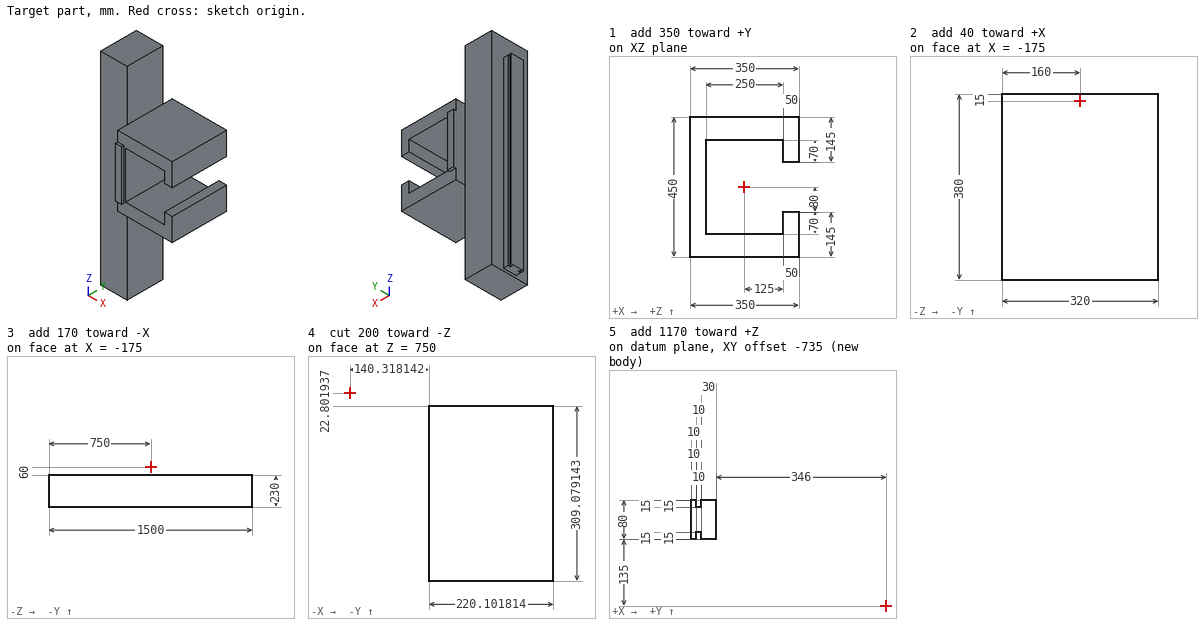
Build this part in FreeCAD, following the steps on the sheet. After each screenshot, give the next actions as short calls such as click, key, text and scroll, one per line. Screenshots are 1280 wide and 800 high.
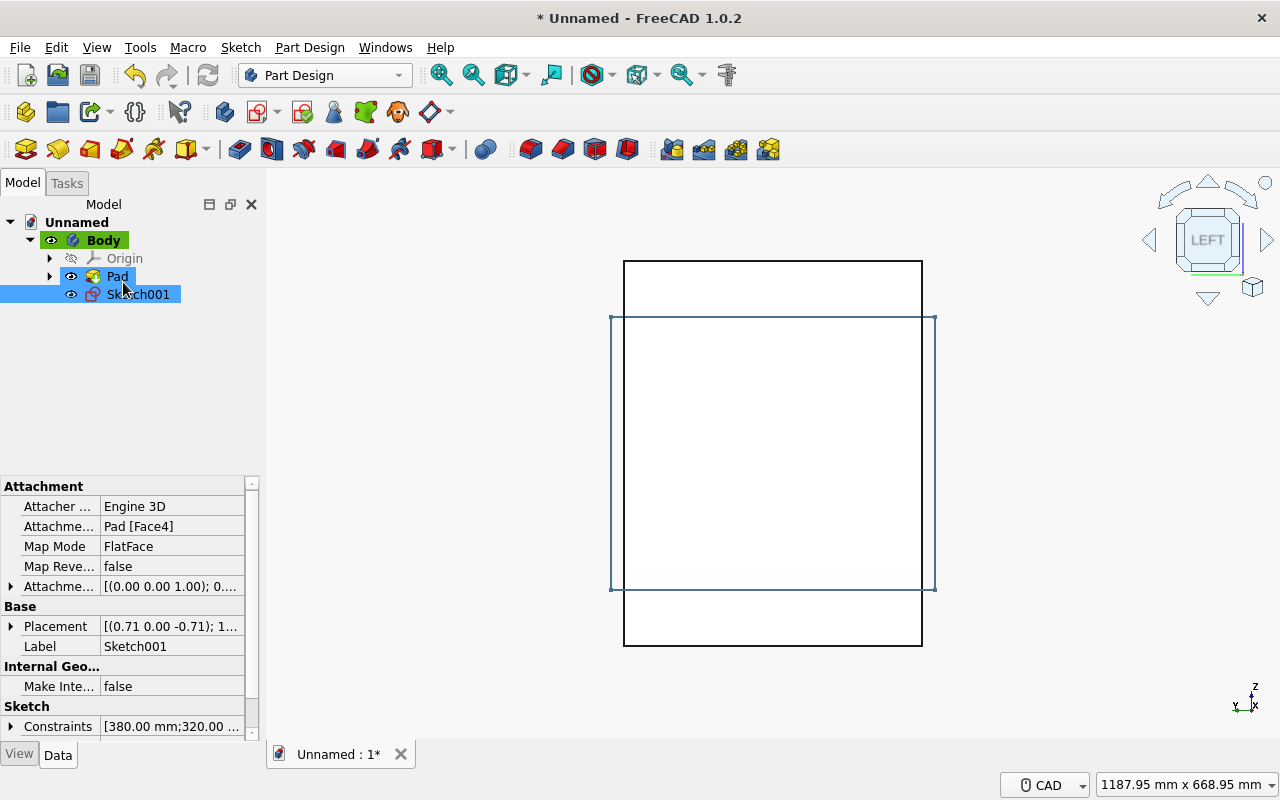
click(26, 150)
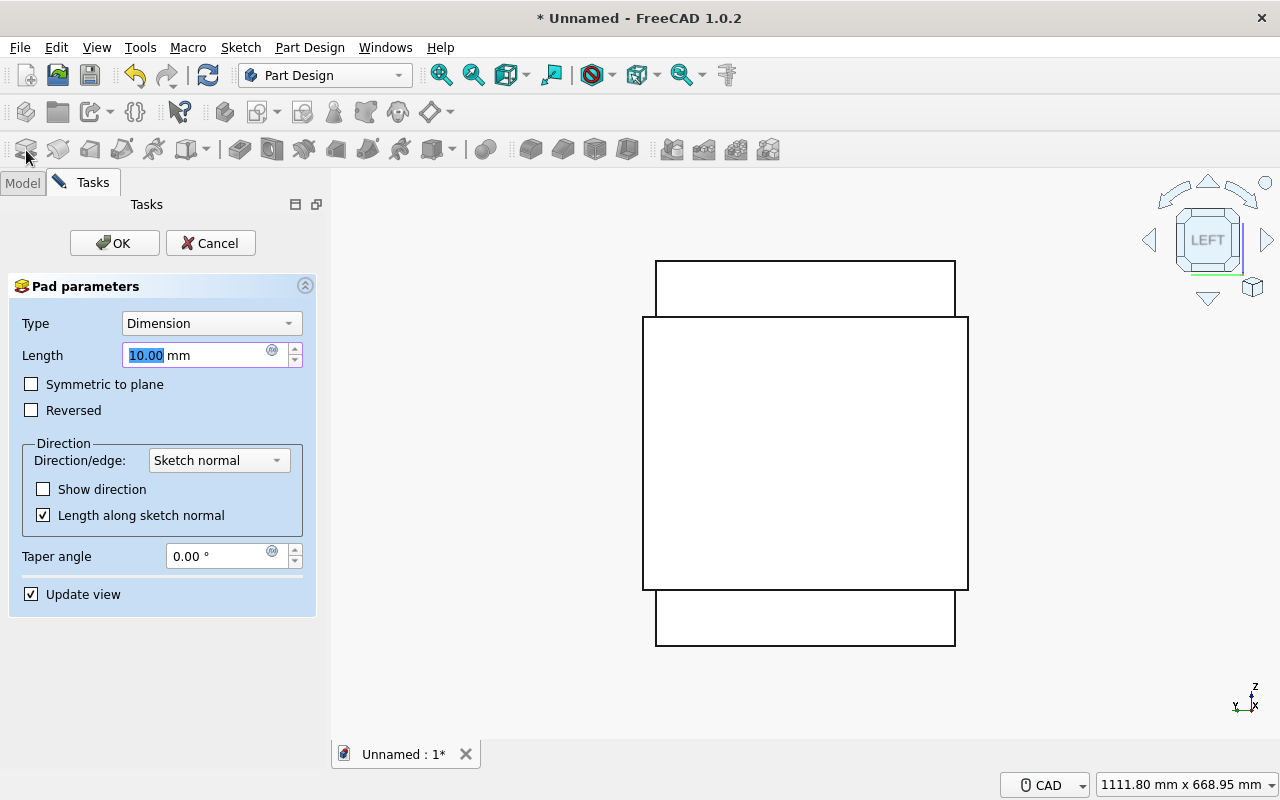
text(40)
key(Tab)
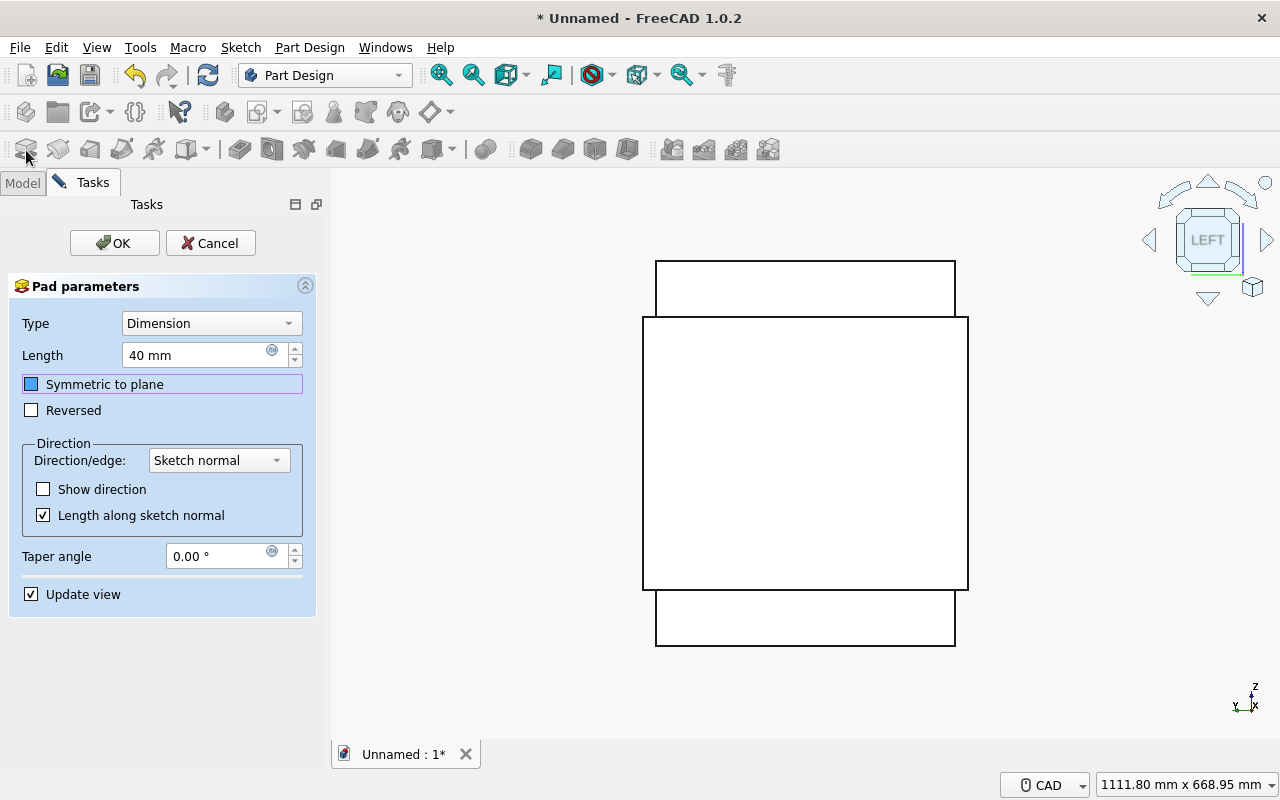
click(30, 410)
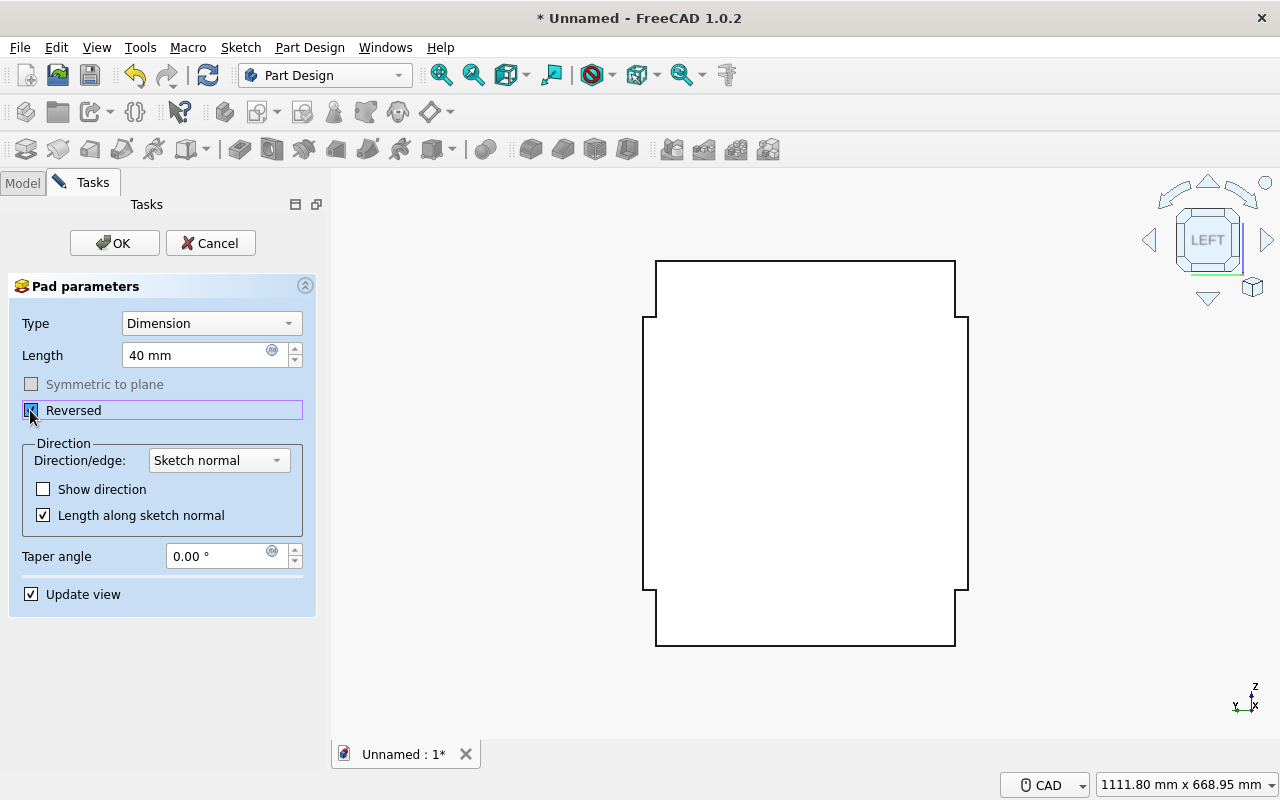
click(115, 243)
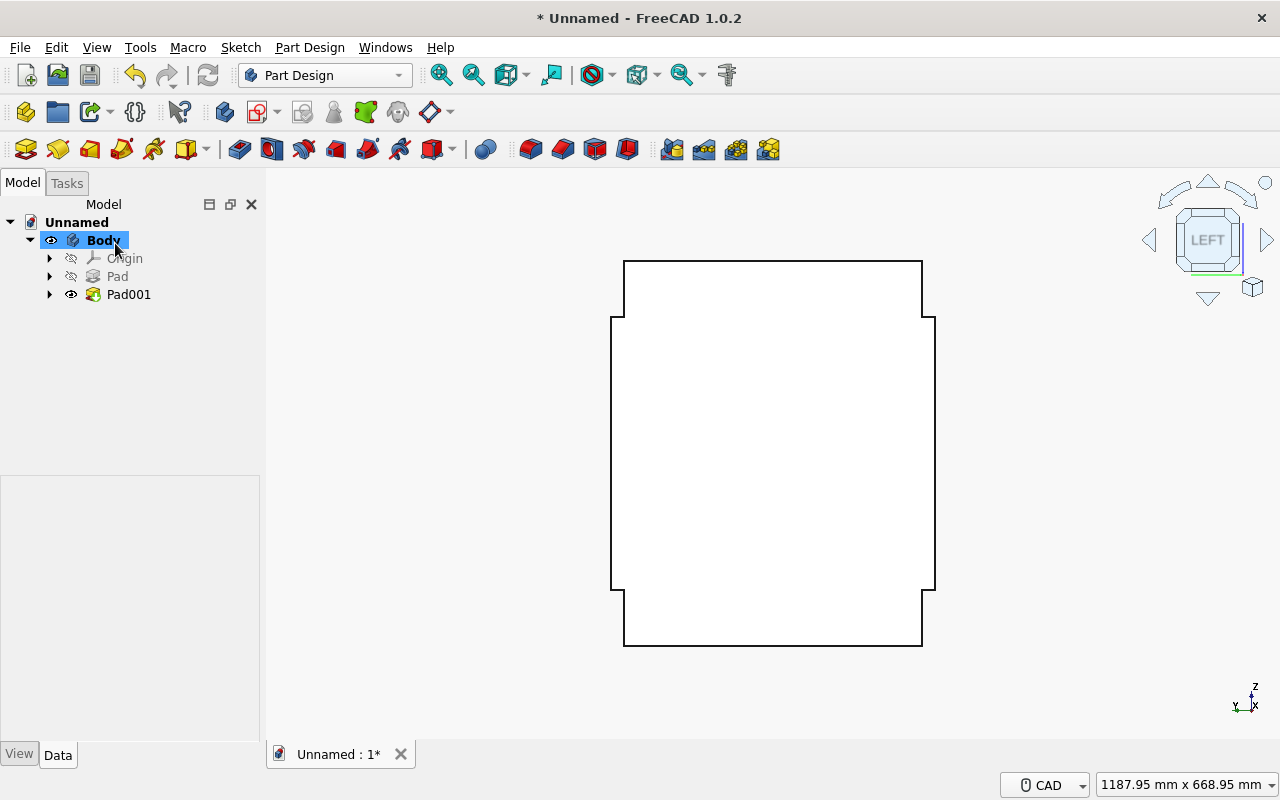
click(773, 453)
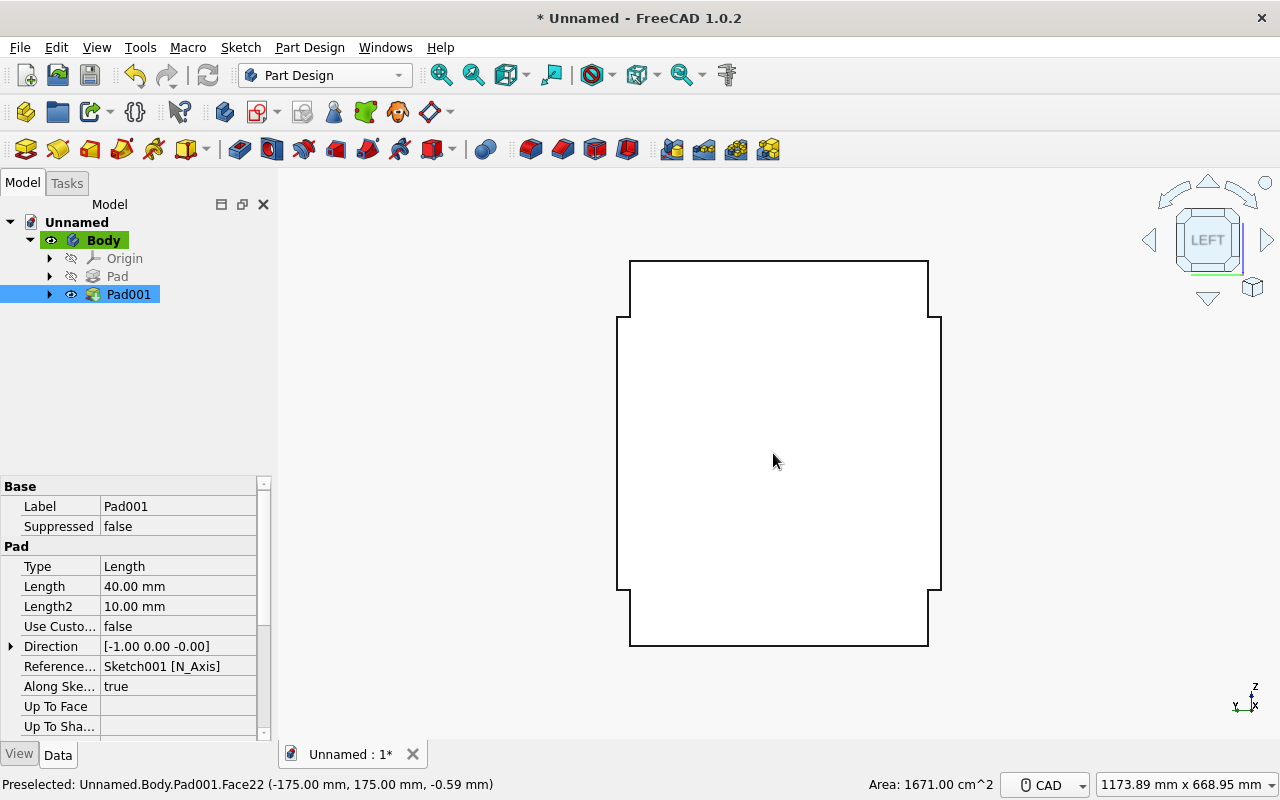
click(258, 112)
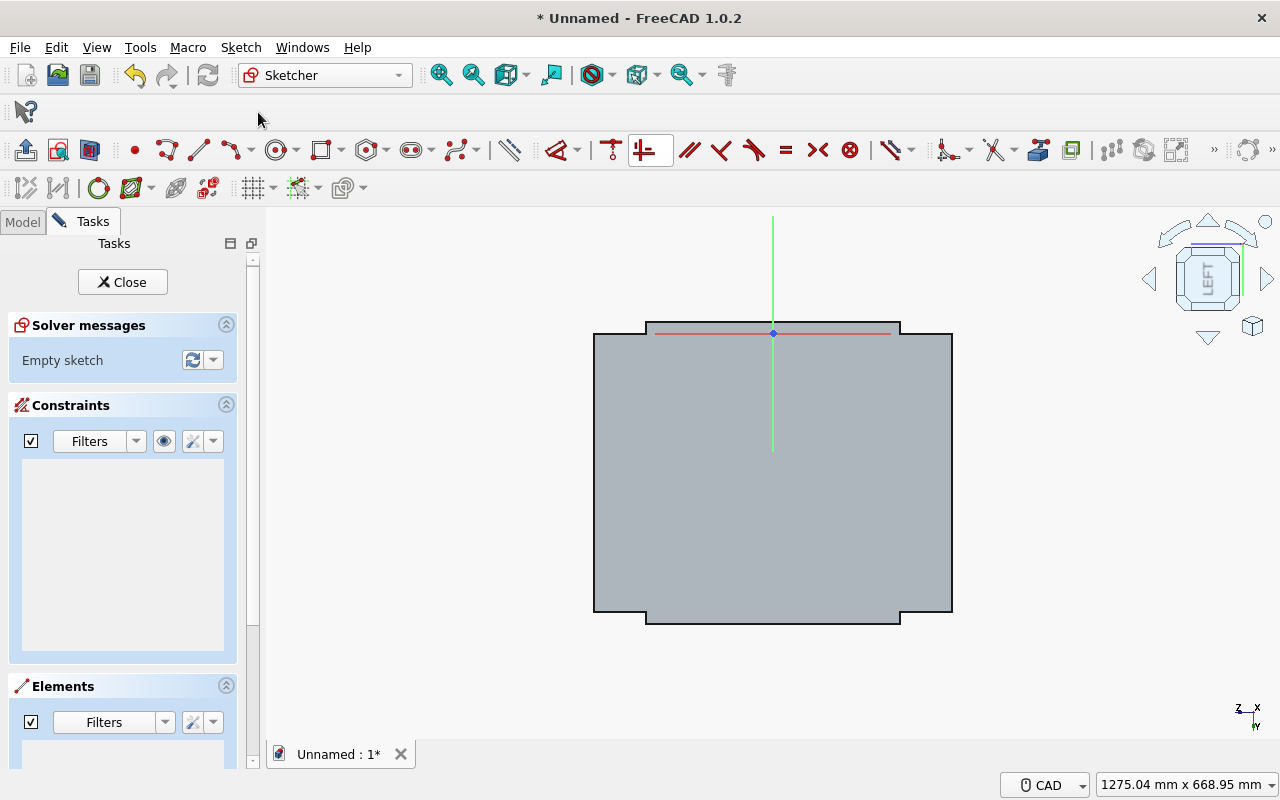
scroll(649, 492, down, 4)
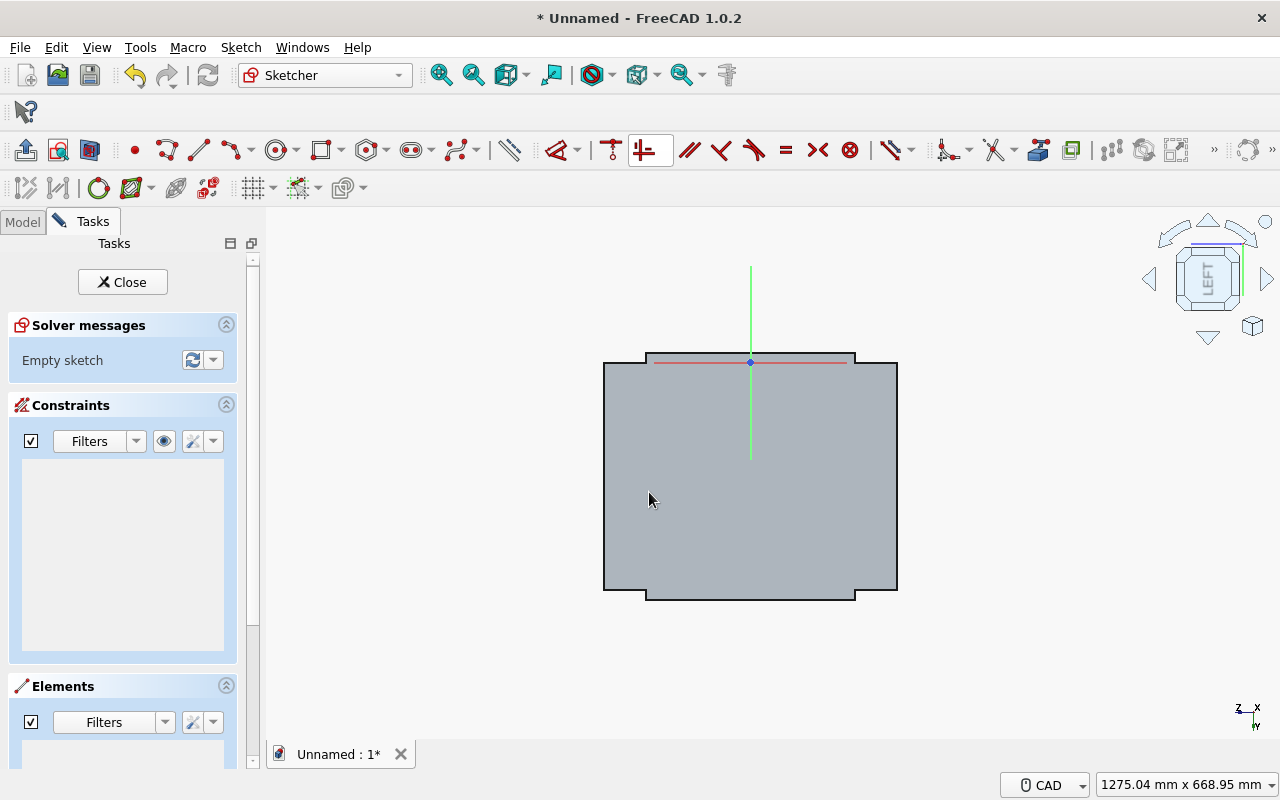
key(g)
key(r)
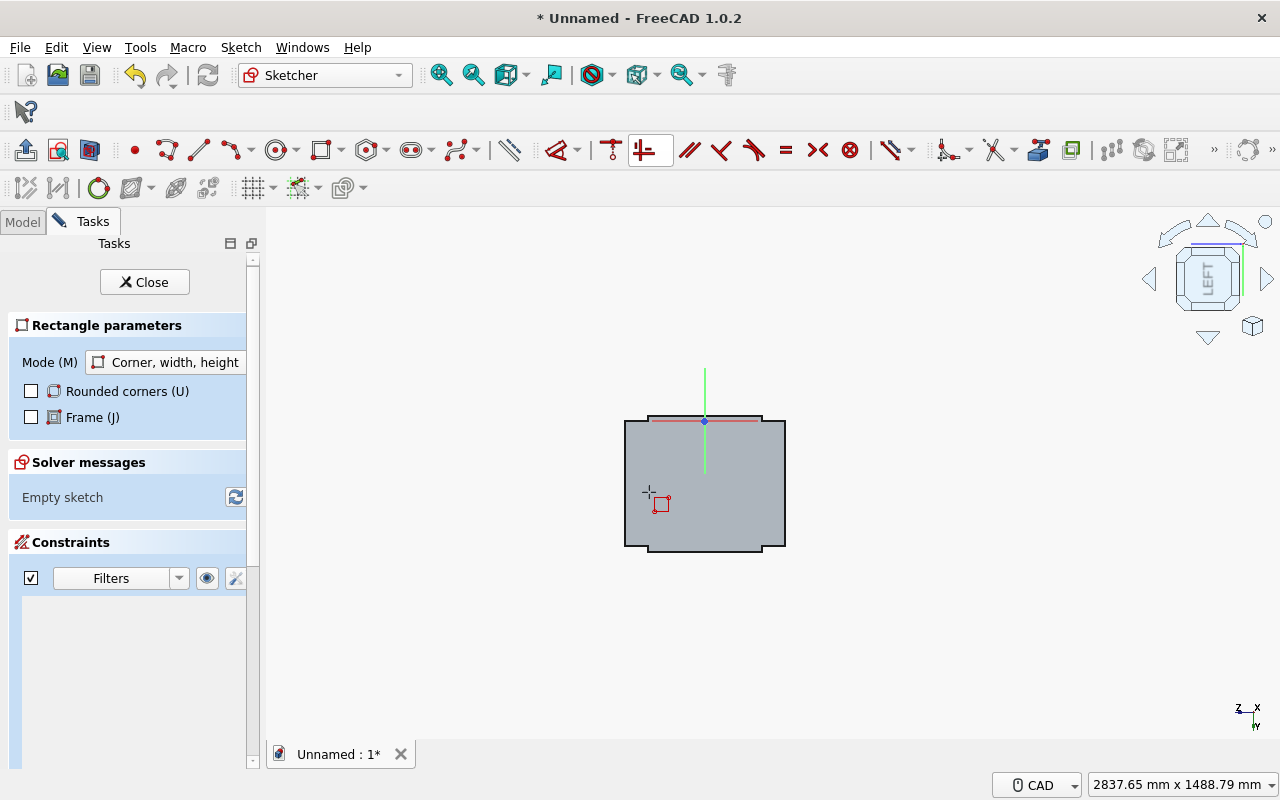
click(437, 443)
move(973, 525)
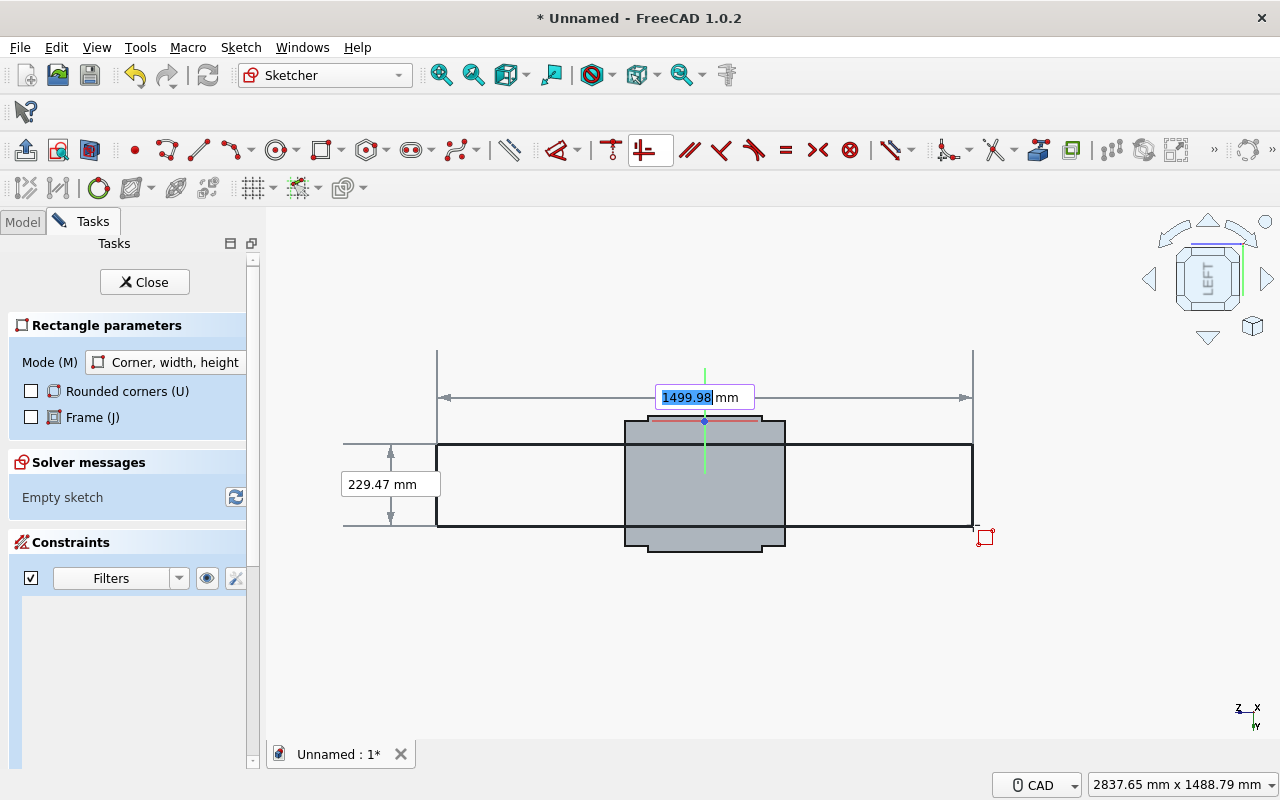
text(1500)
key(Tab)
text(230)
key(Return)
key(Escape)